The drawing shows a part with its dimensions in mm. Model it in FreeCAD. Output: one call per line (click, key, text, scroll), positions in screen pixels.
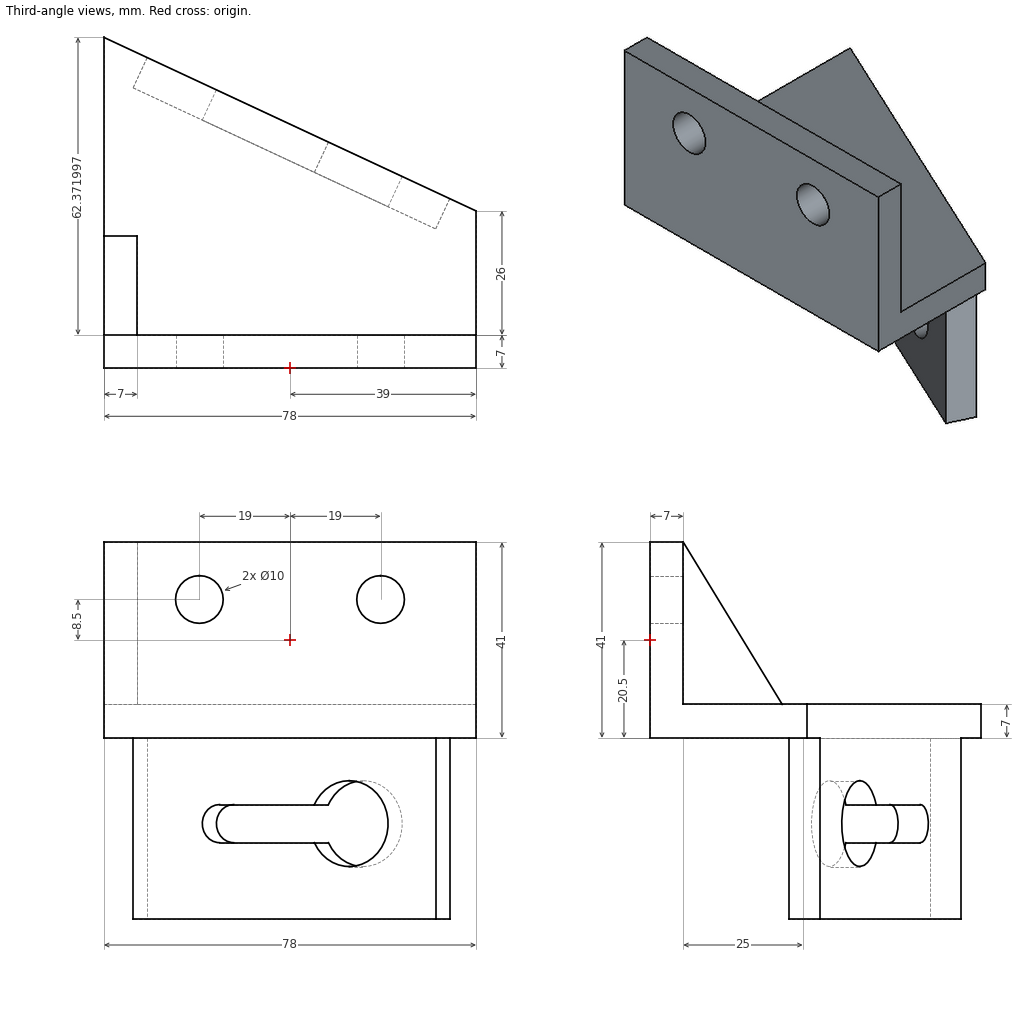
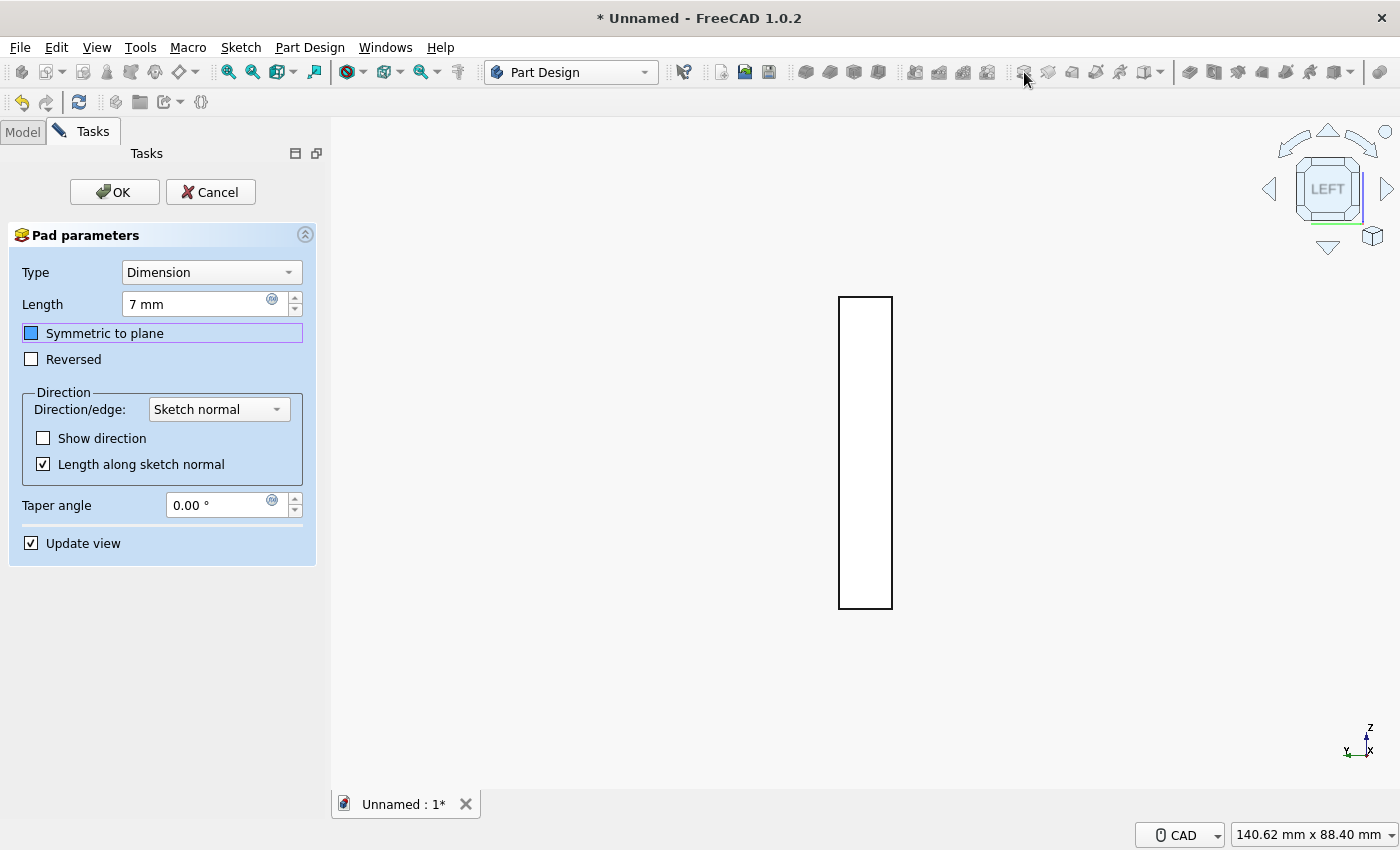
click(30, 359)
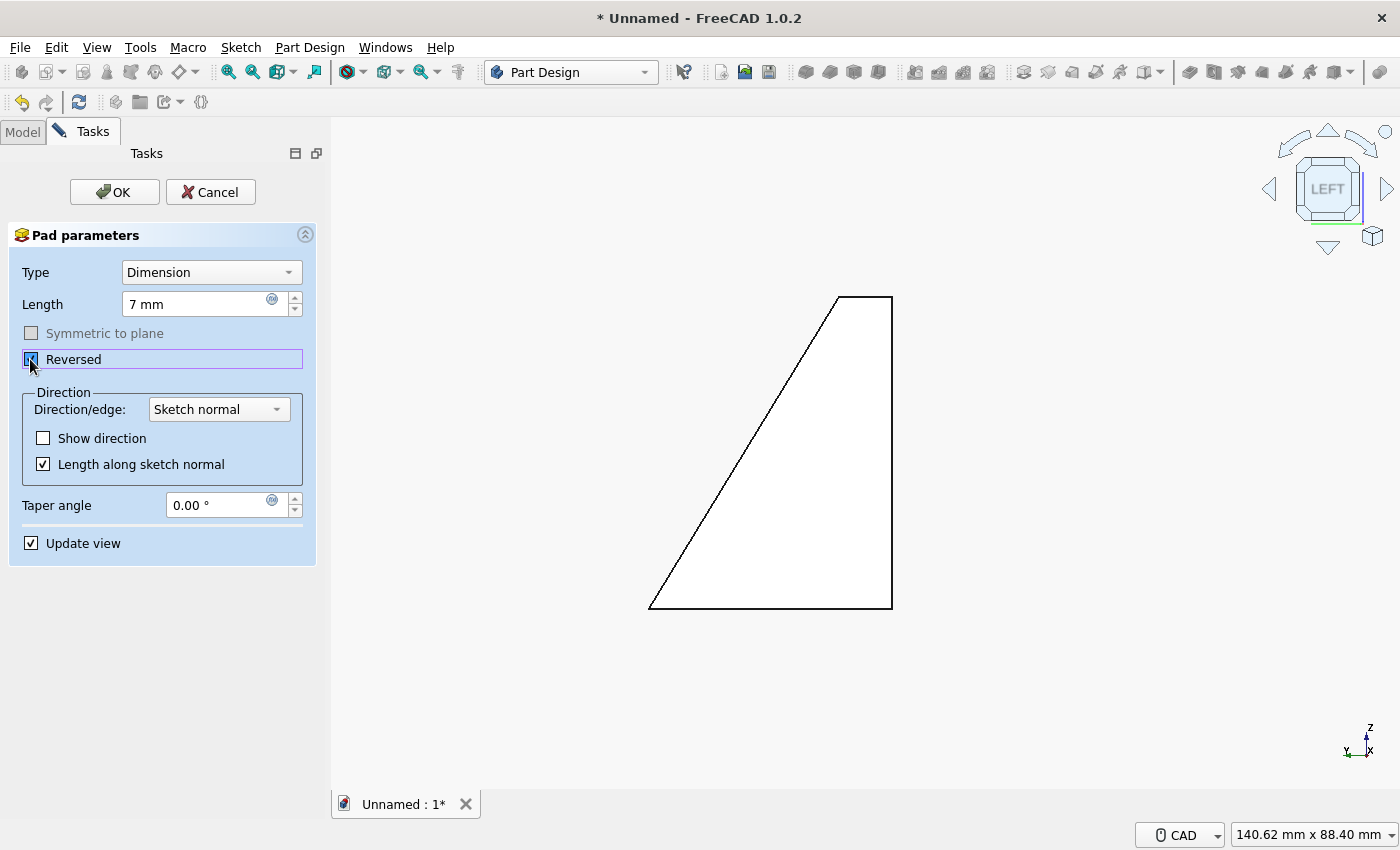
click(115, 192)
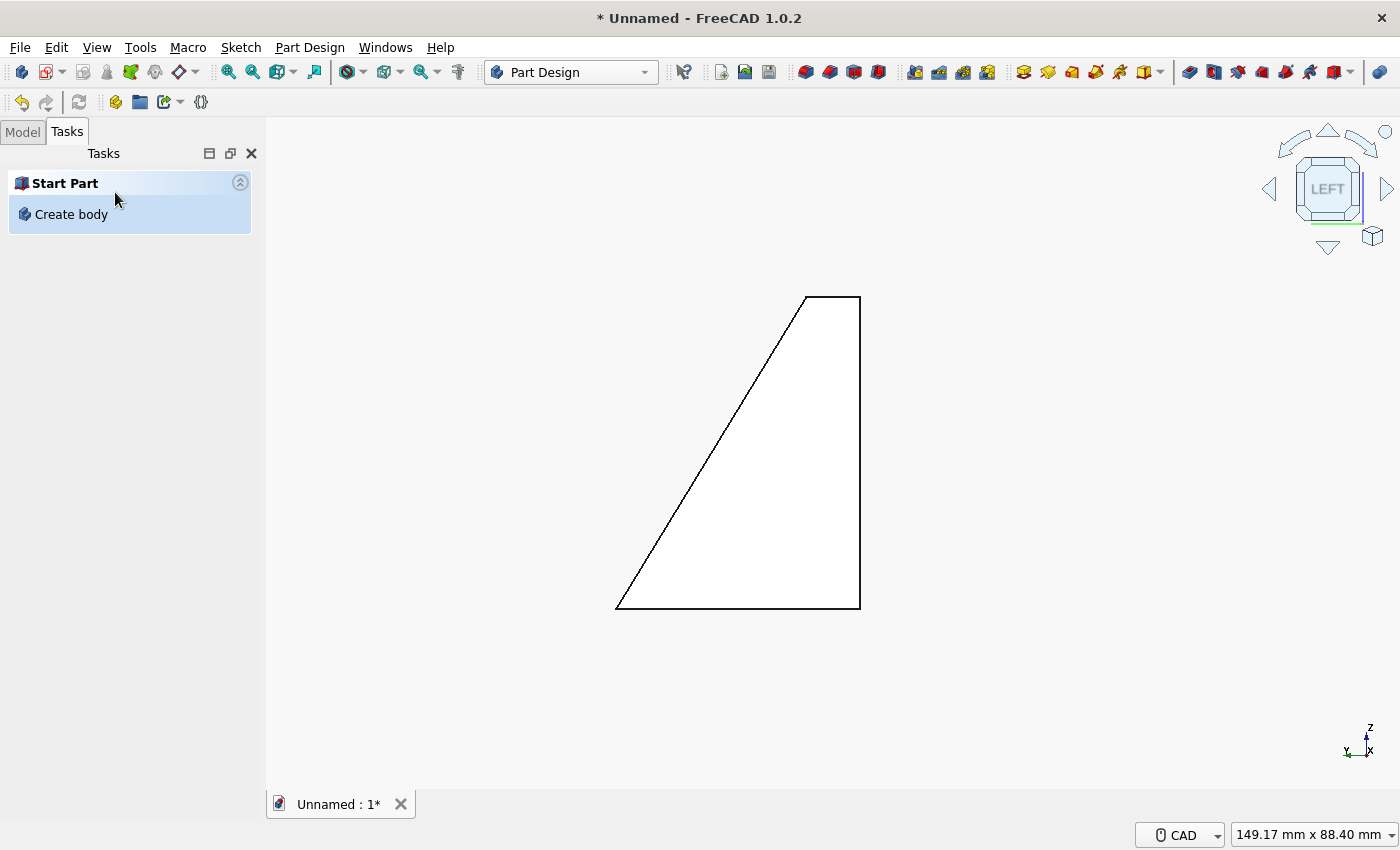
key(5)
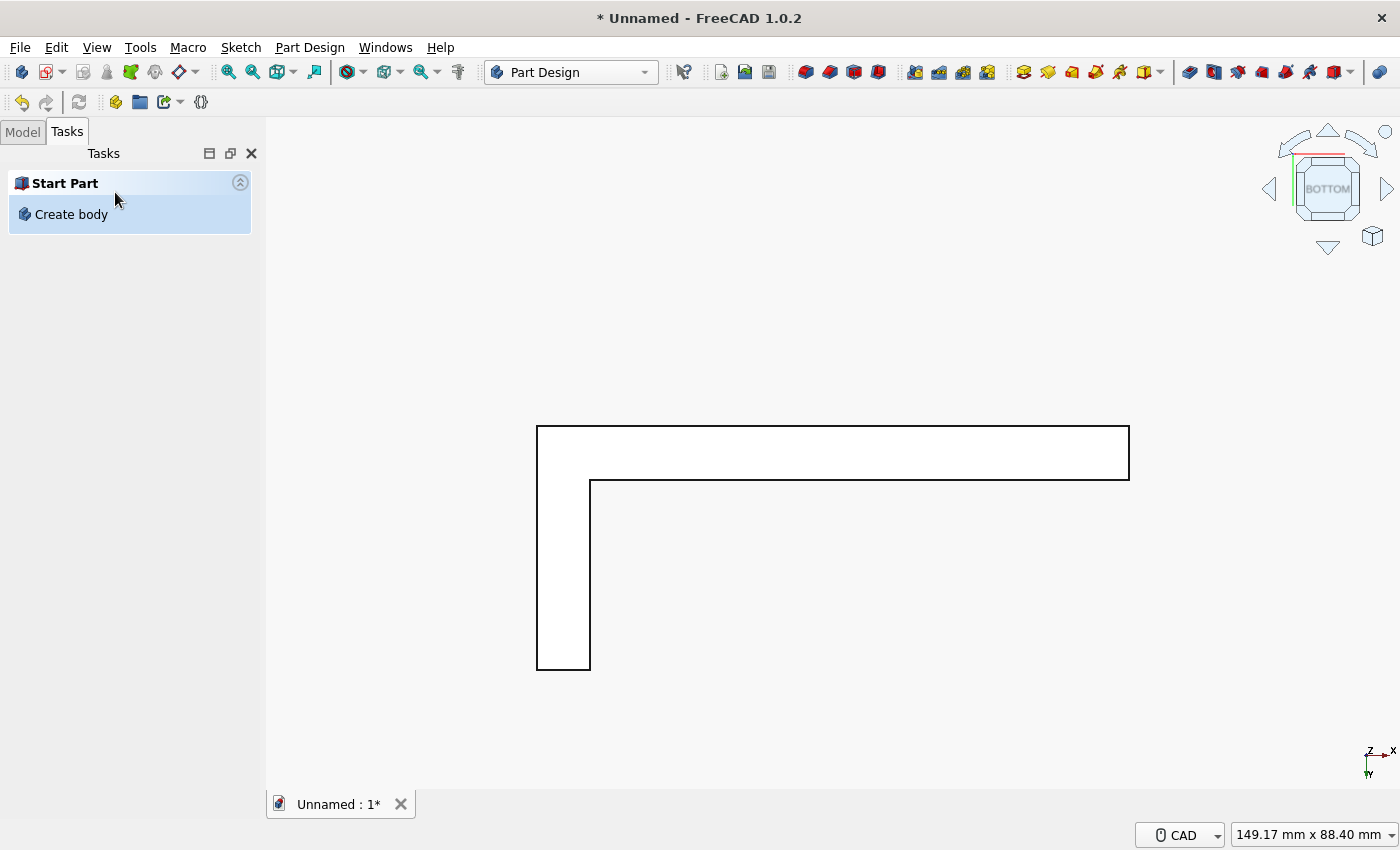
click(1087, 443)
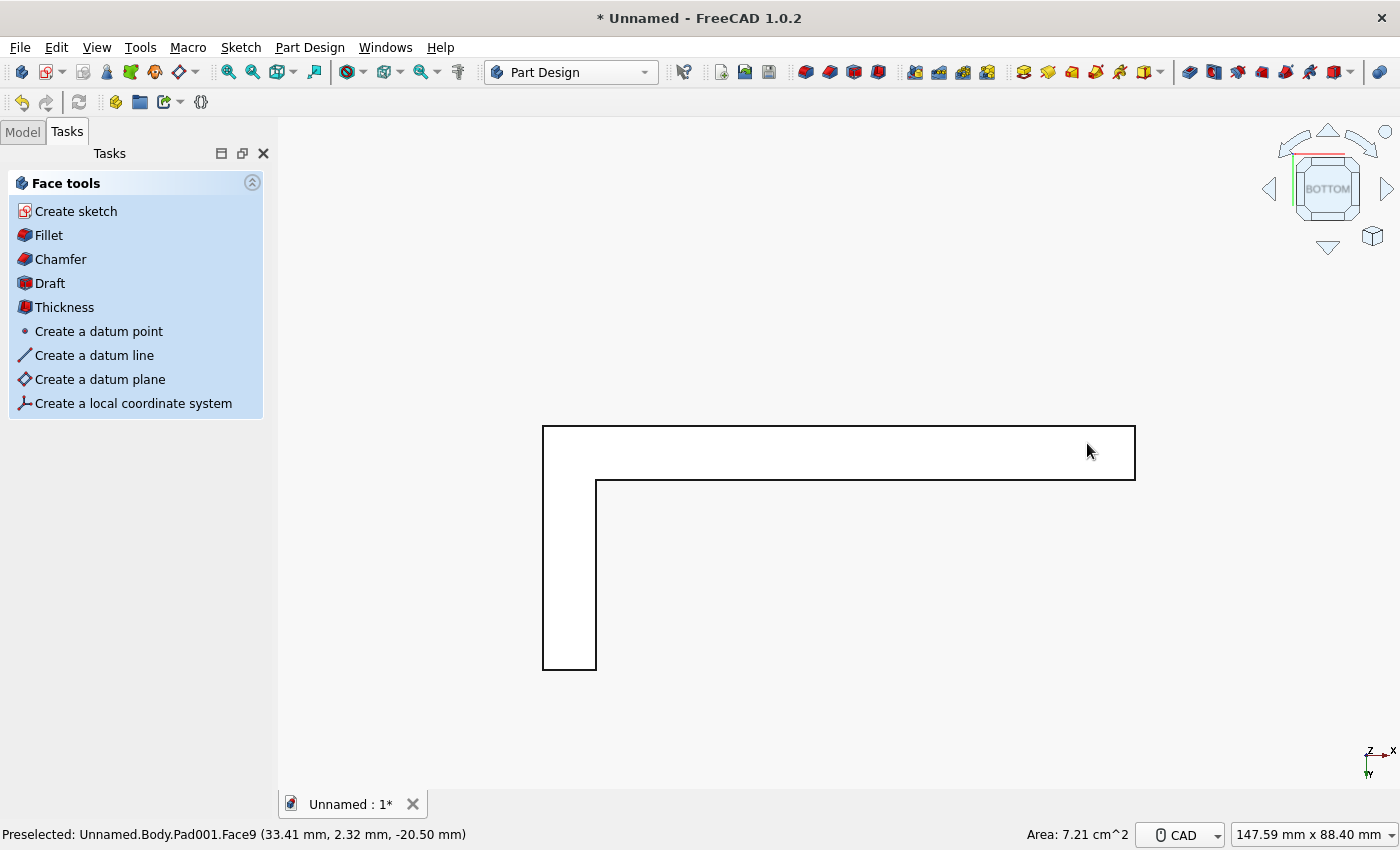
click(46, 72)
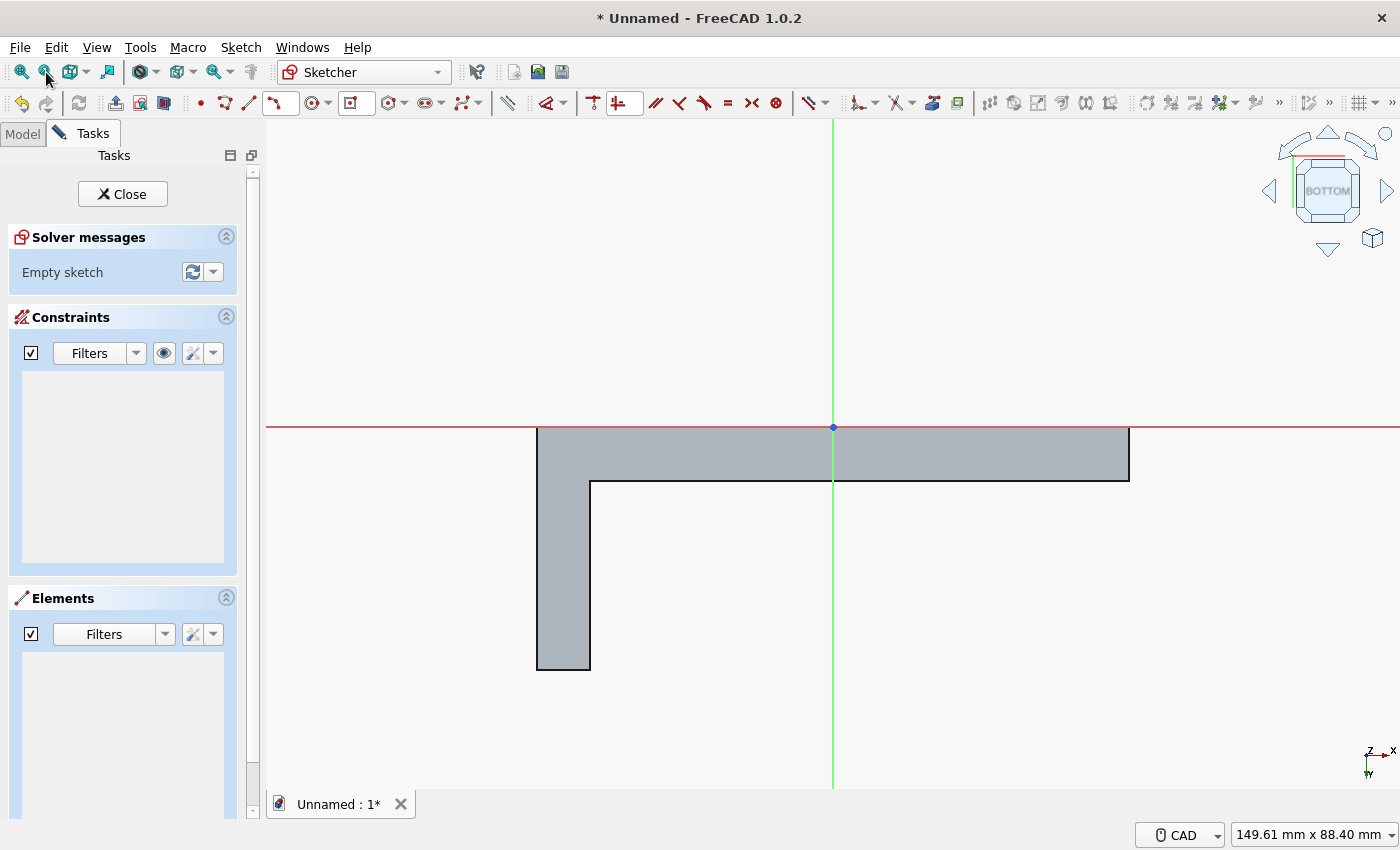
scroll(625, 147, down, 2)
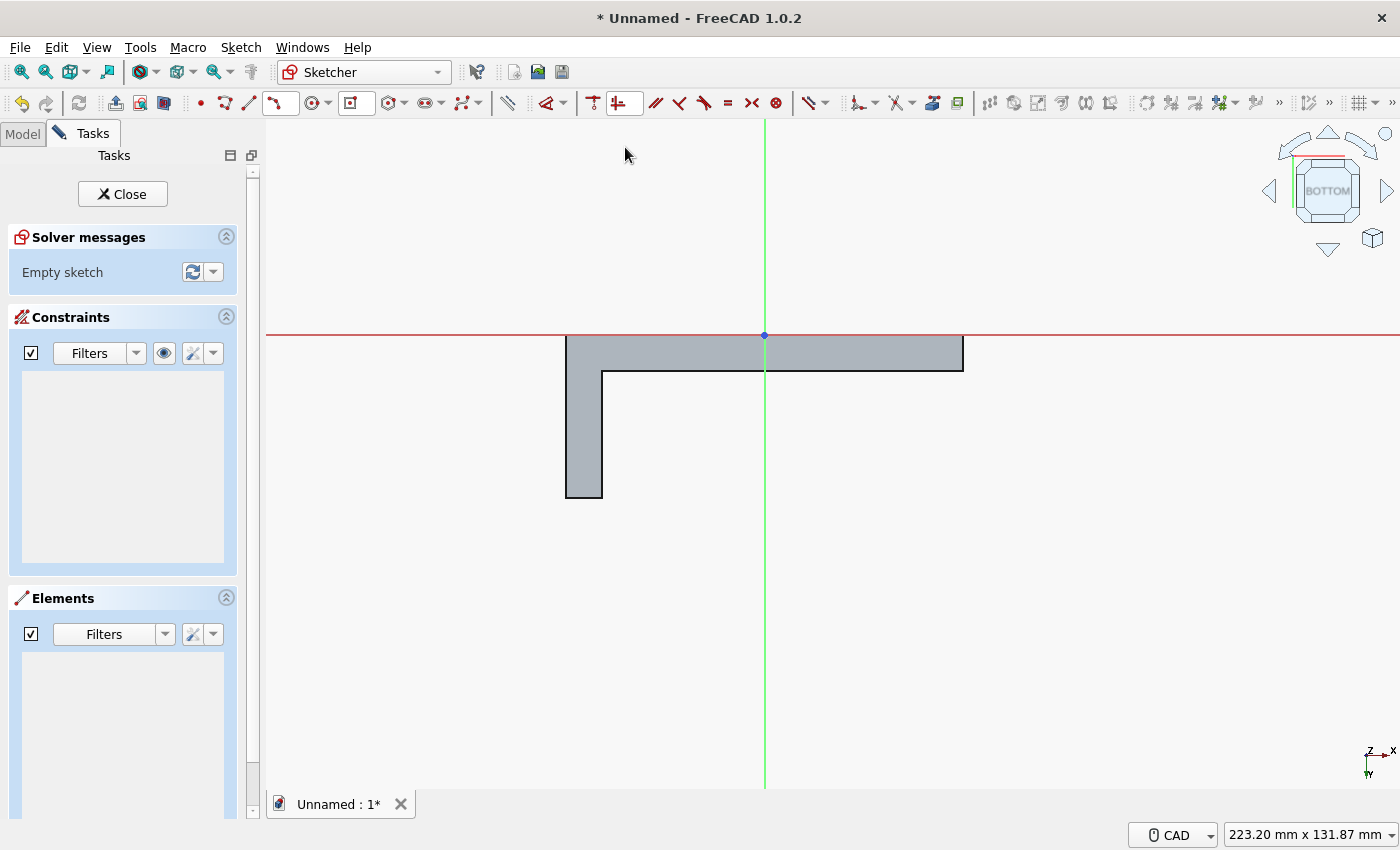
click(226, 104)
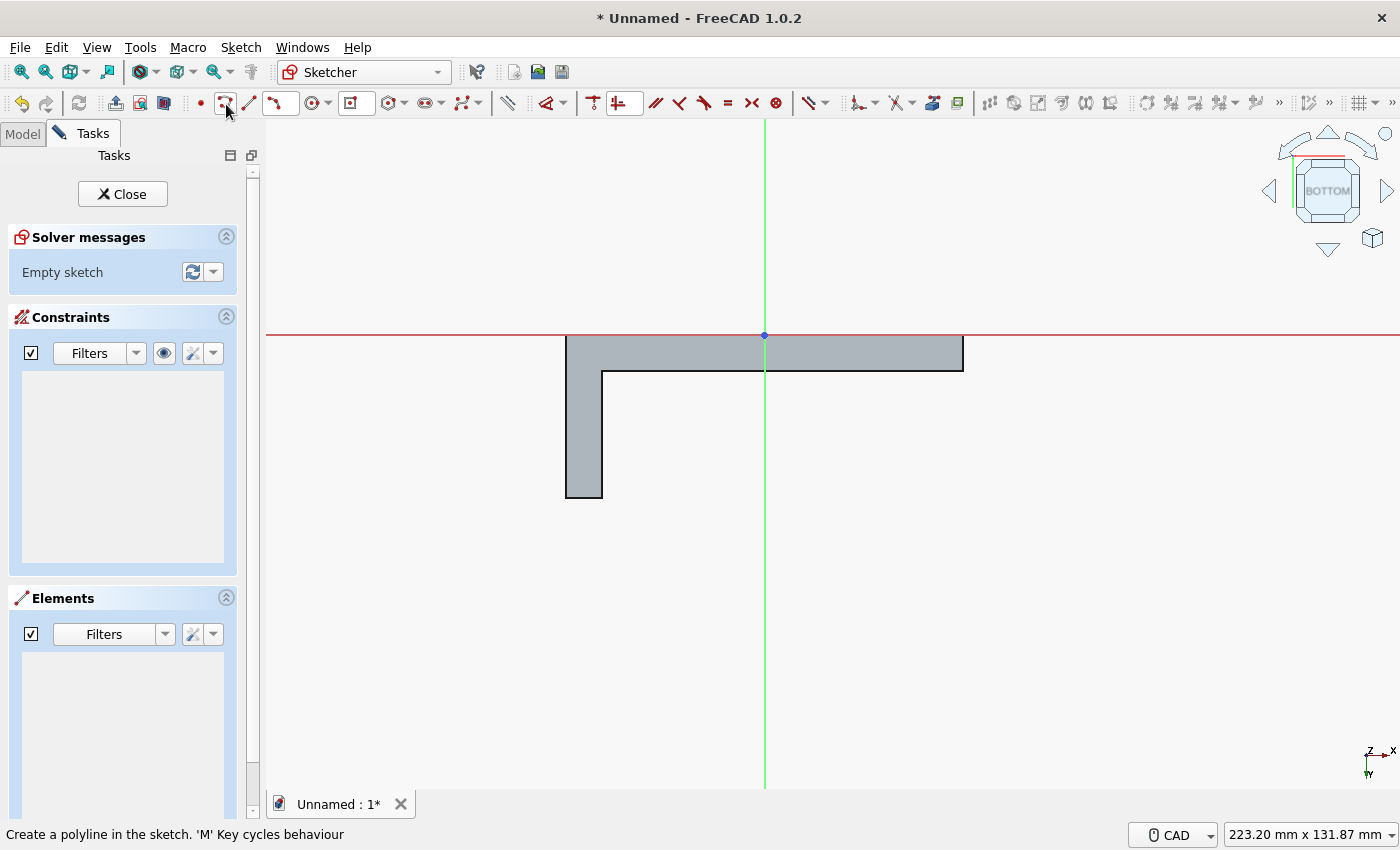
click(963, 371)
click(566, 371)
click(566, 687)
click(963, 503)
click(963, 372)
key(Escape)
key(Escape)